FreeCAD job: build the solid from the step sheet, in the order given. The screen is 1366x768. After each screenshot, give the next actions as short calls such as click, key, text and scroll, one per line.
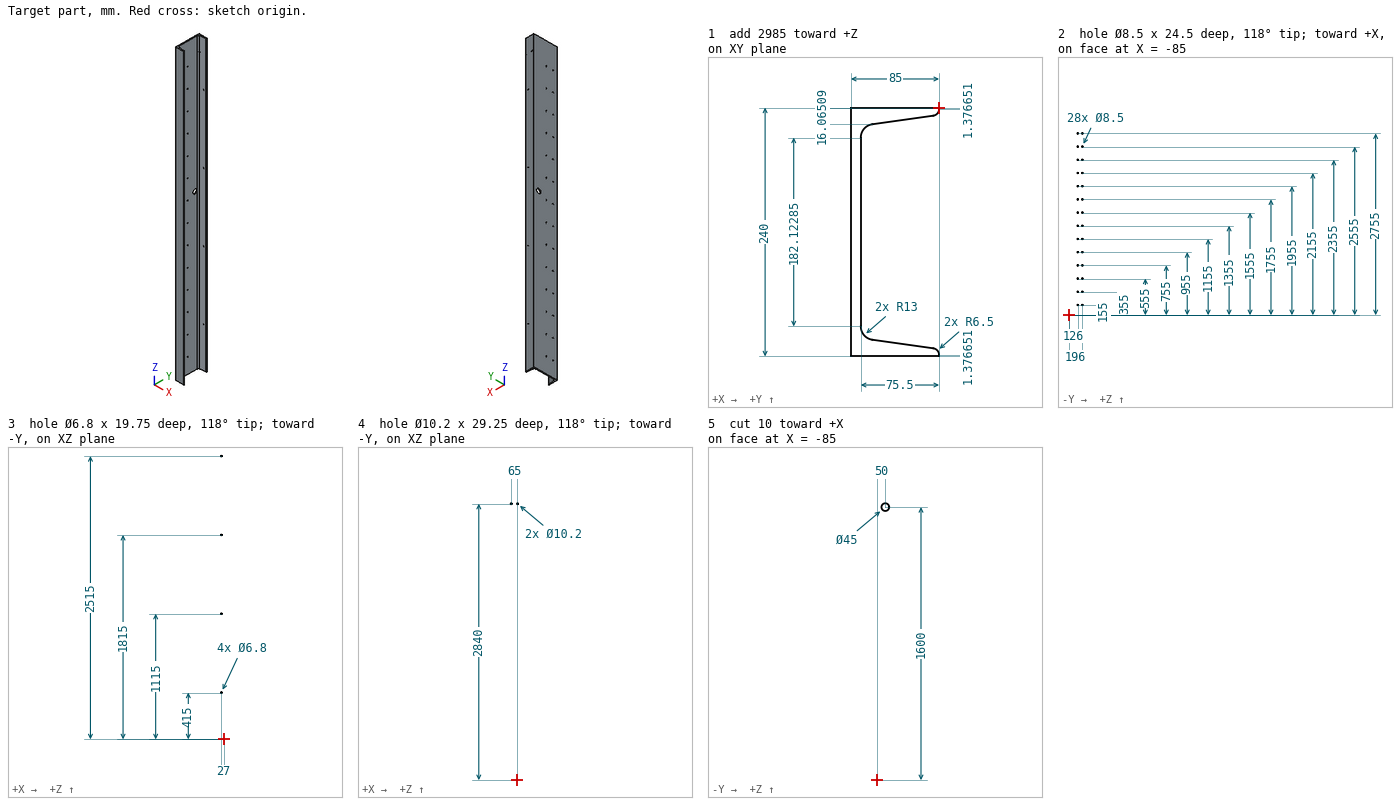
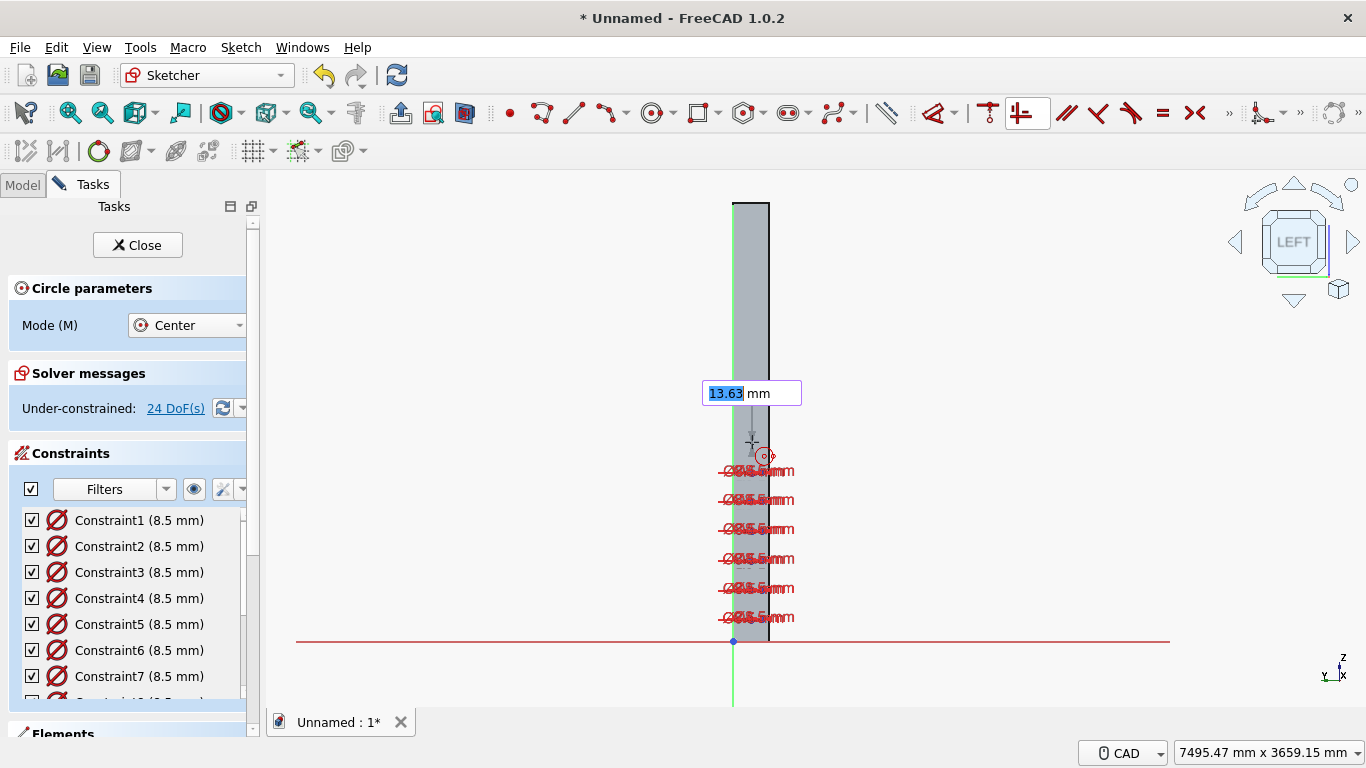
text(8.5)
key(Return)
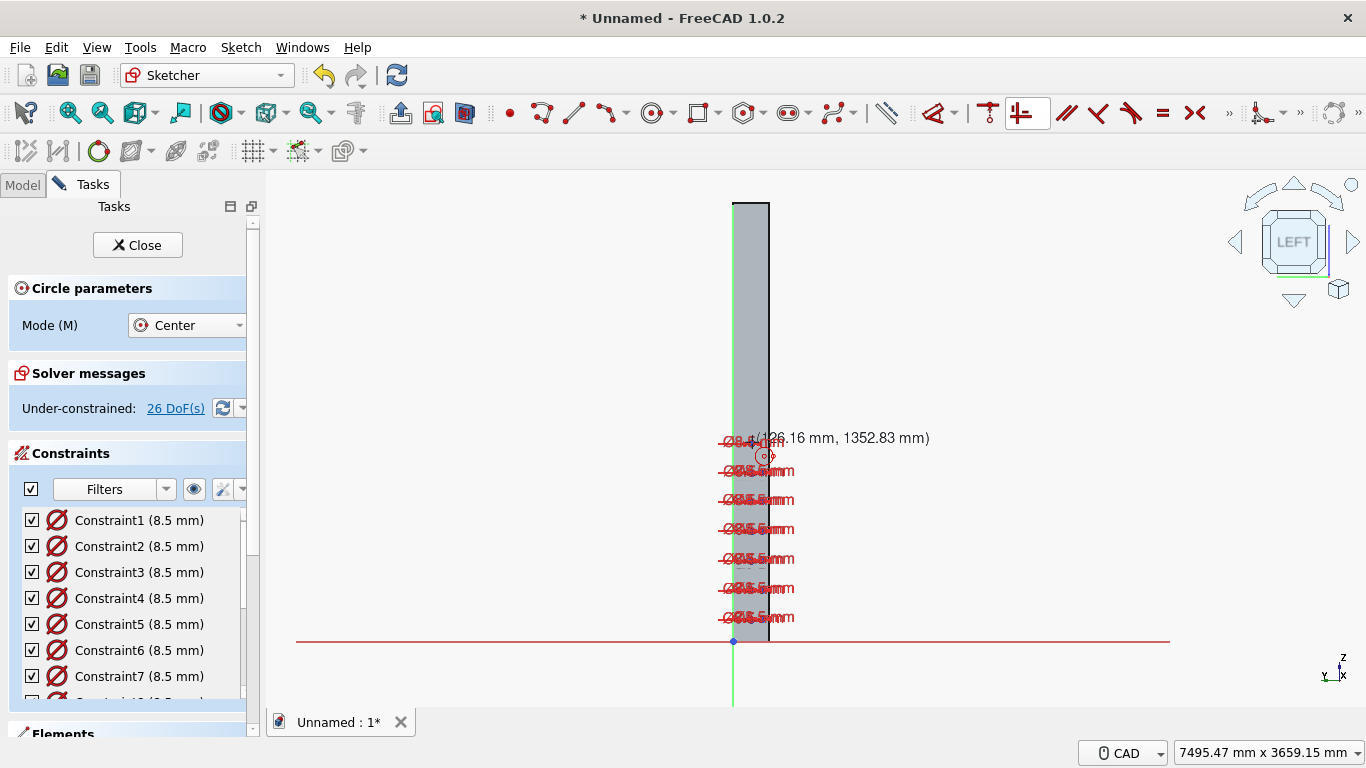
scroll(762, 443, up, 18)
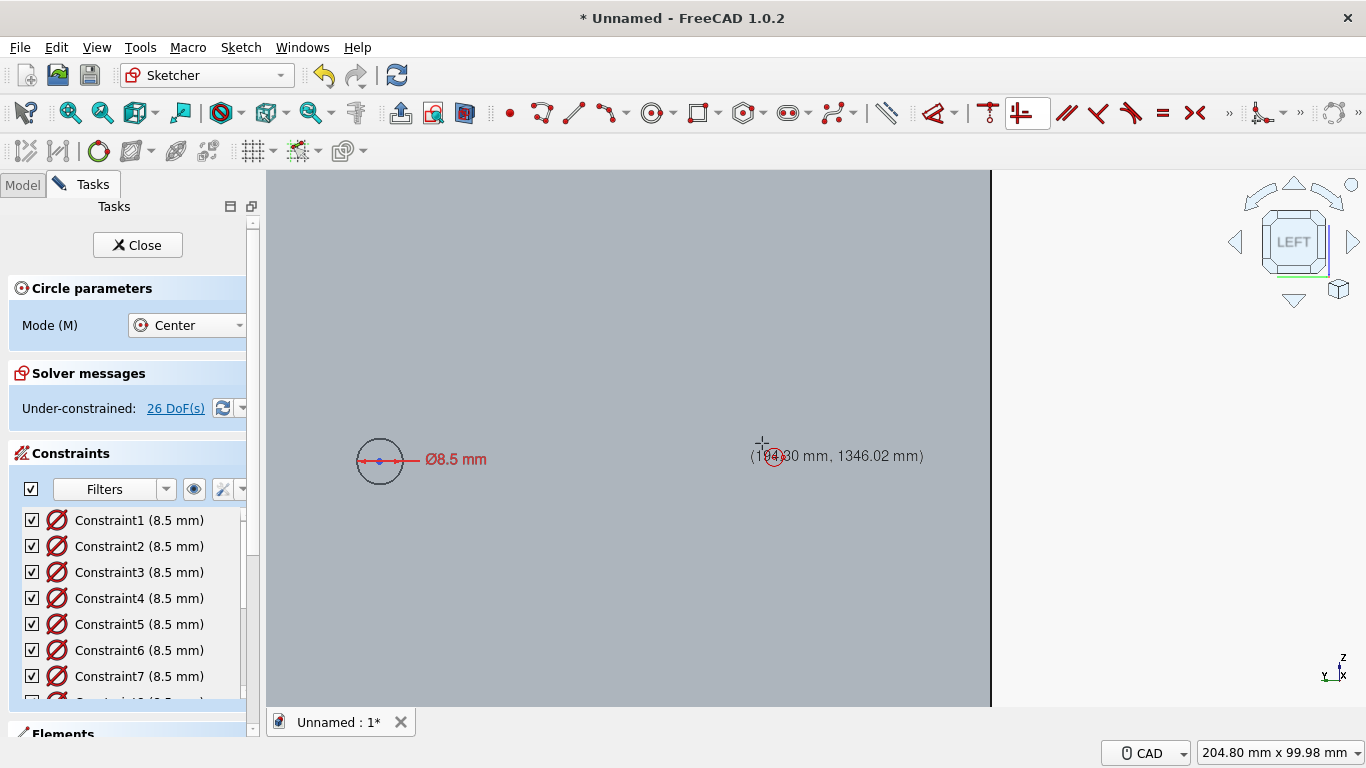
scroll(762, 443, down, 18)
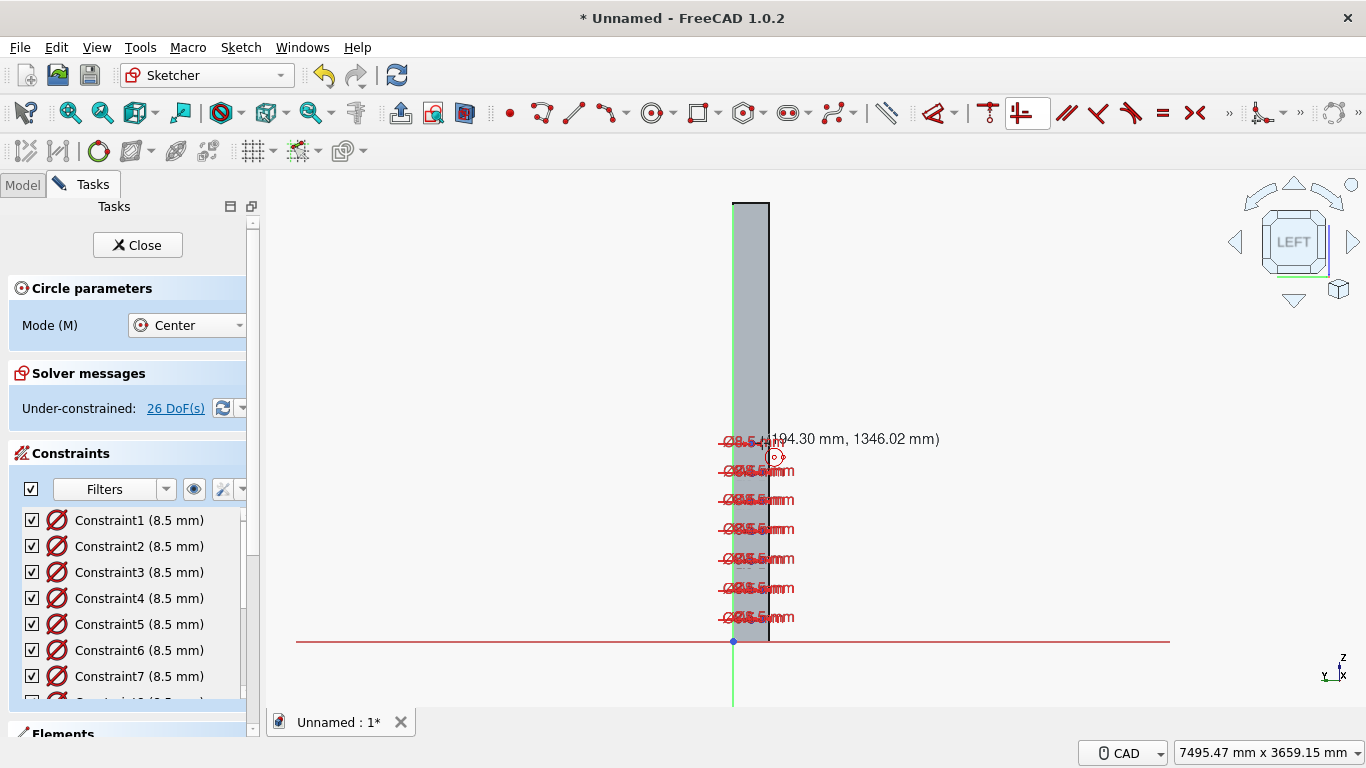
scroll(762, 443, up, 3)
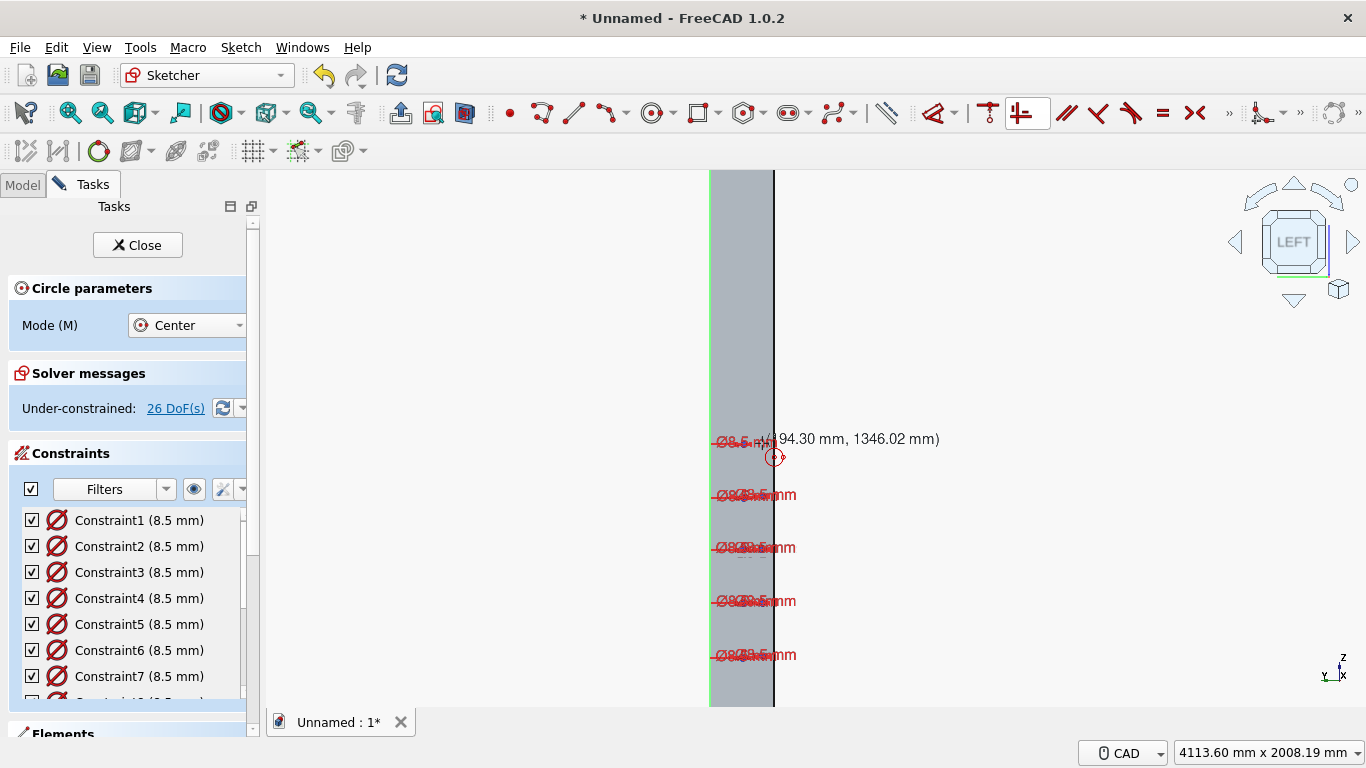
click(762, 442)
move(763, 441)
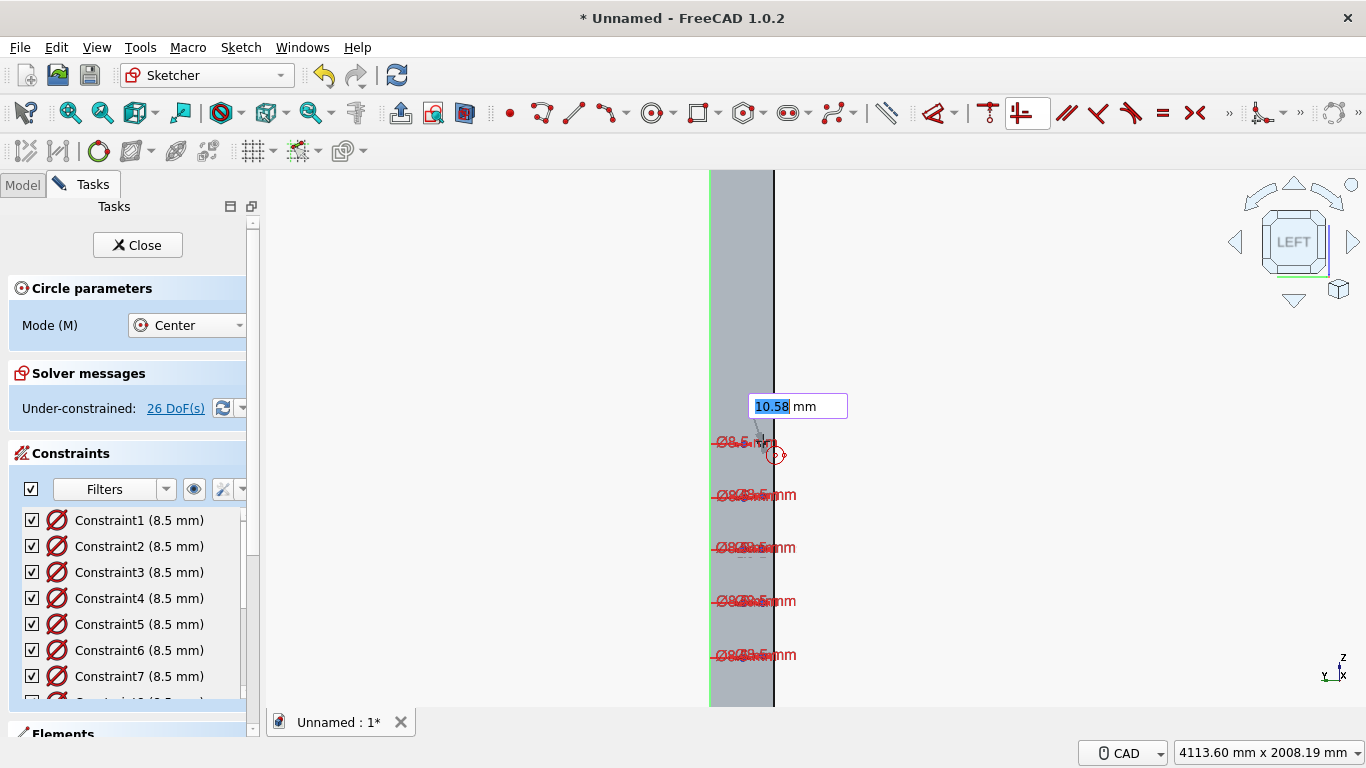
text(8.5)
key(Return)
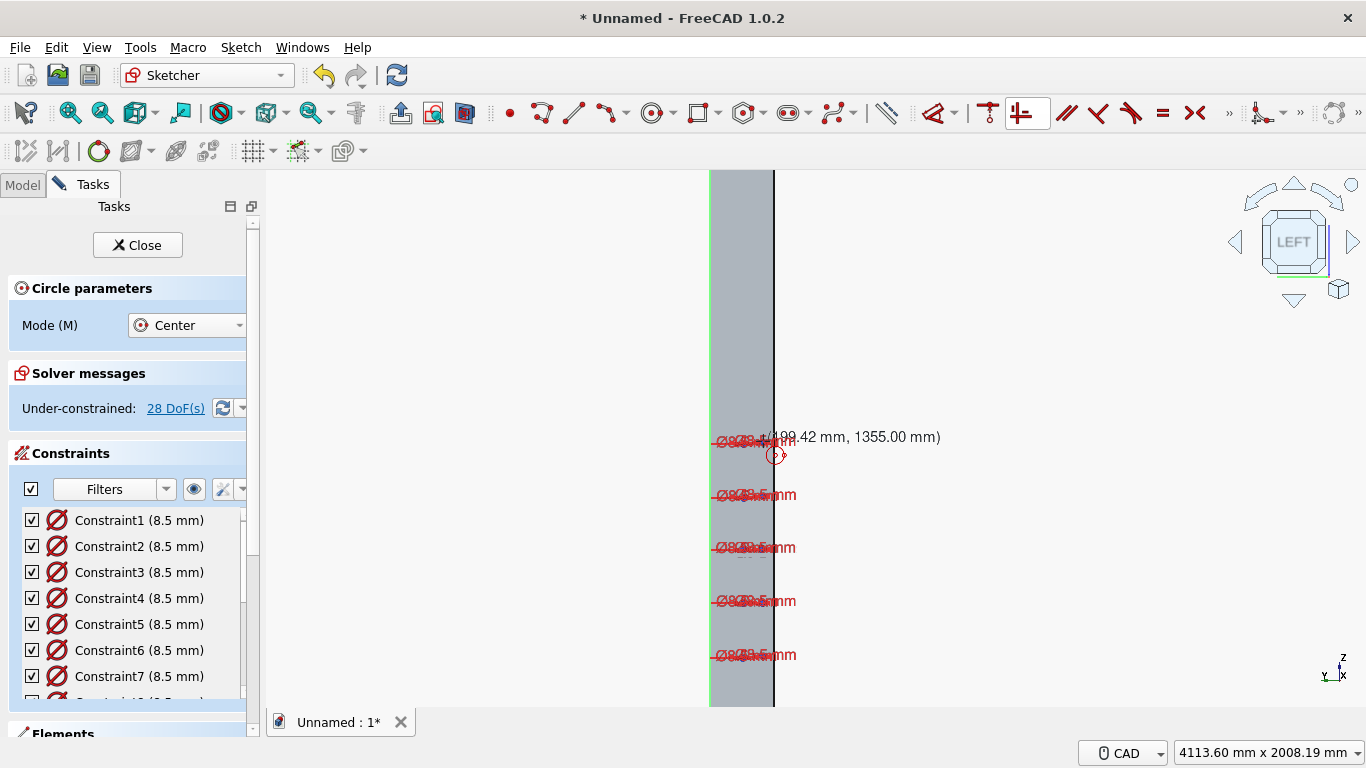
scroll(762, 389, up, 15)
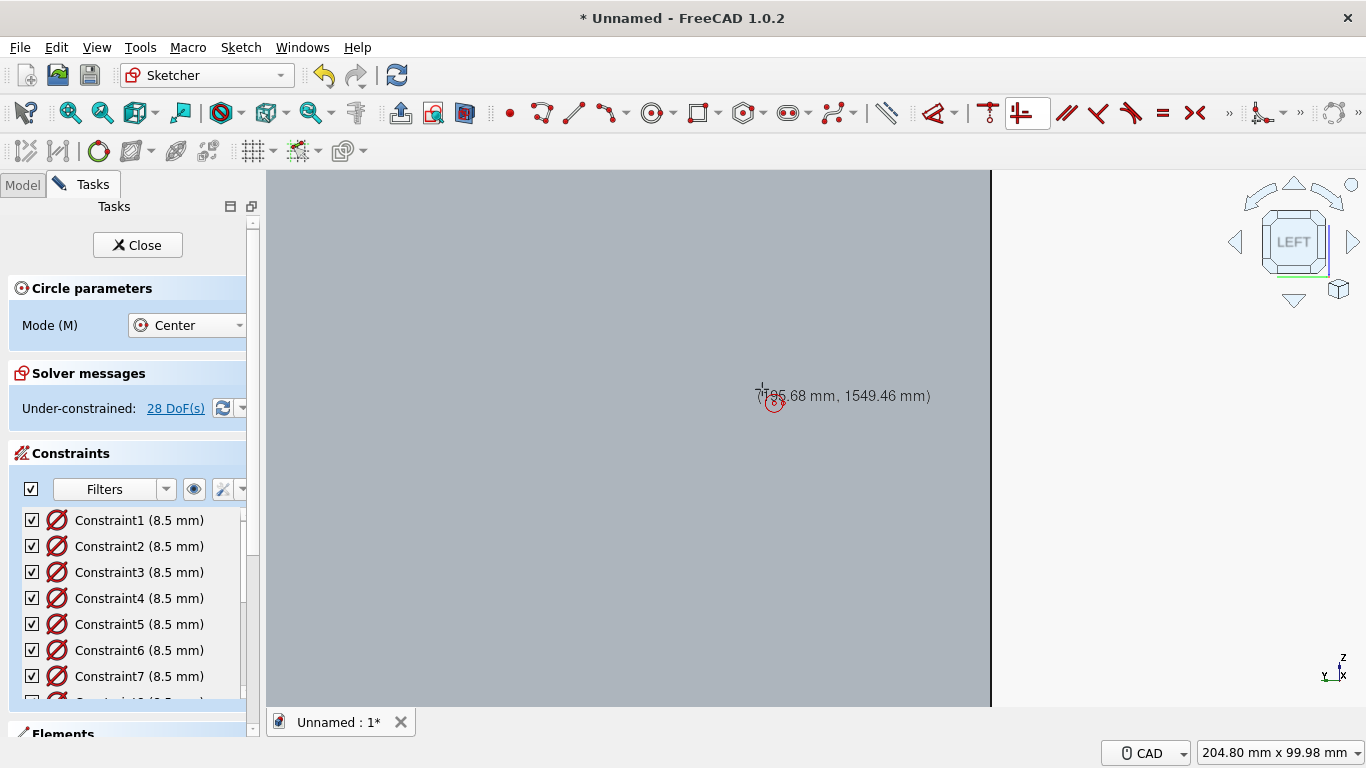
scroll(762, 414, down, 18)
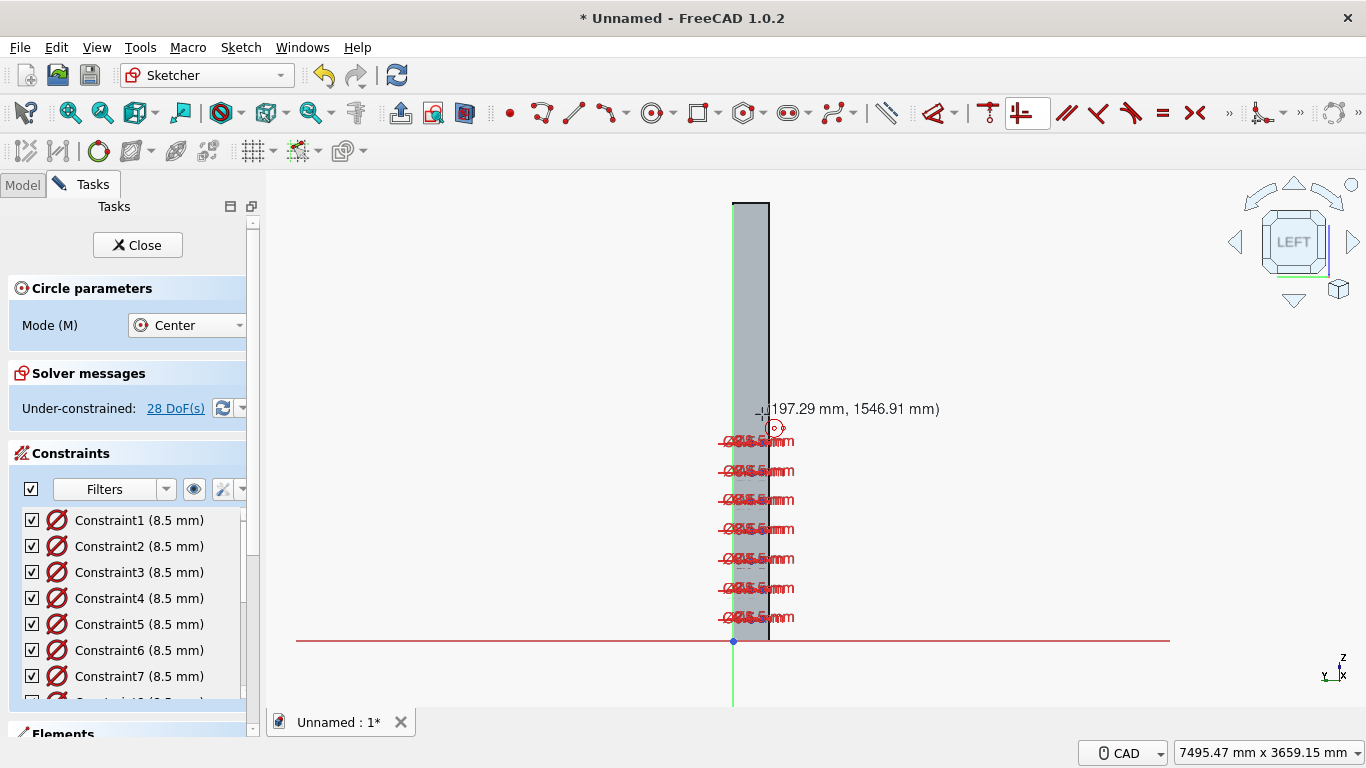
click(762, 413)
move(763, 413)